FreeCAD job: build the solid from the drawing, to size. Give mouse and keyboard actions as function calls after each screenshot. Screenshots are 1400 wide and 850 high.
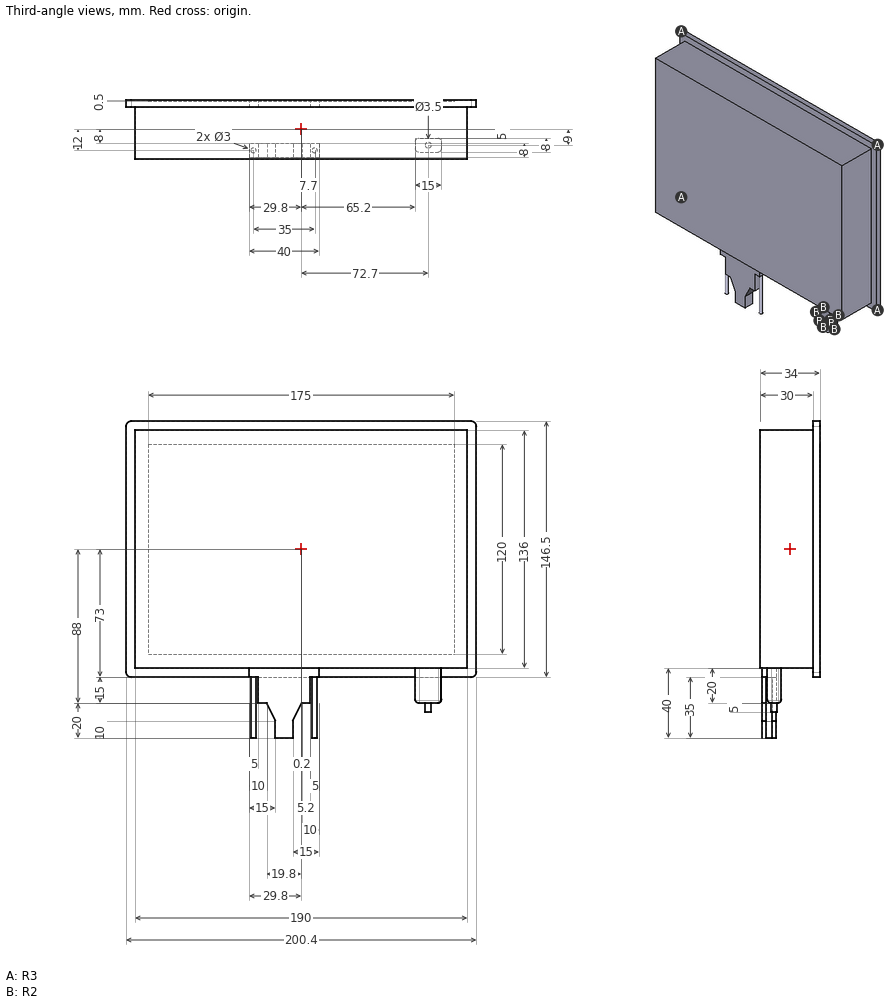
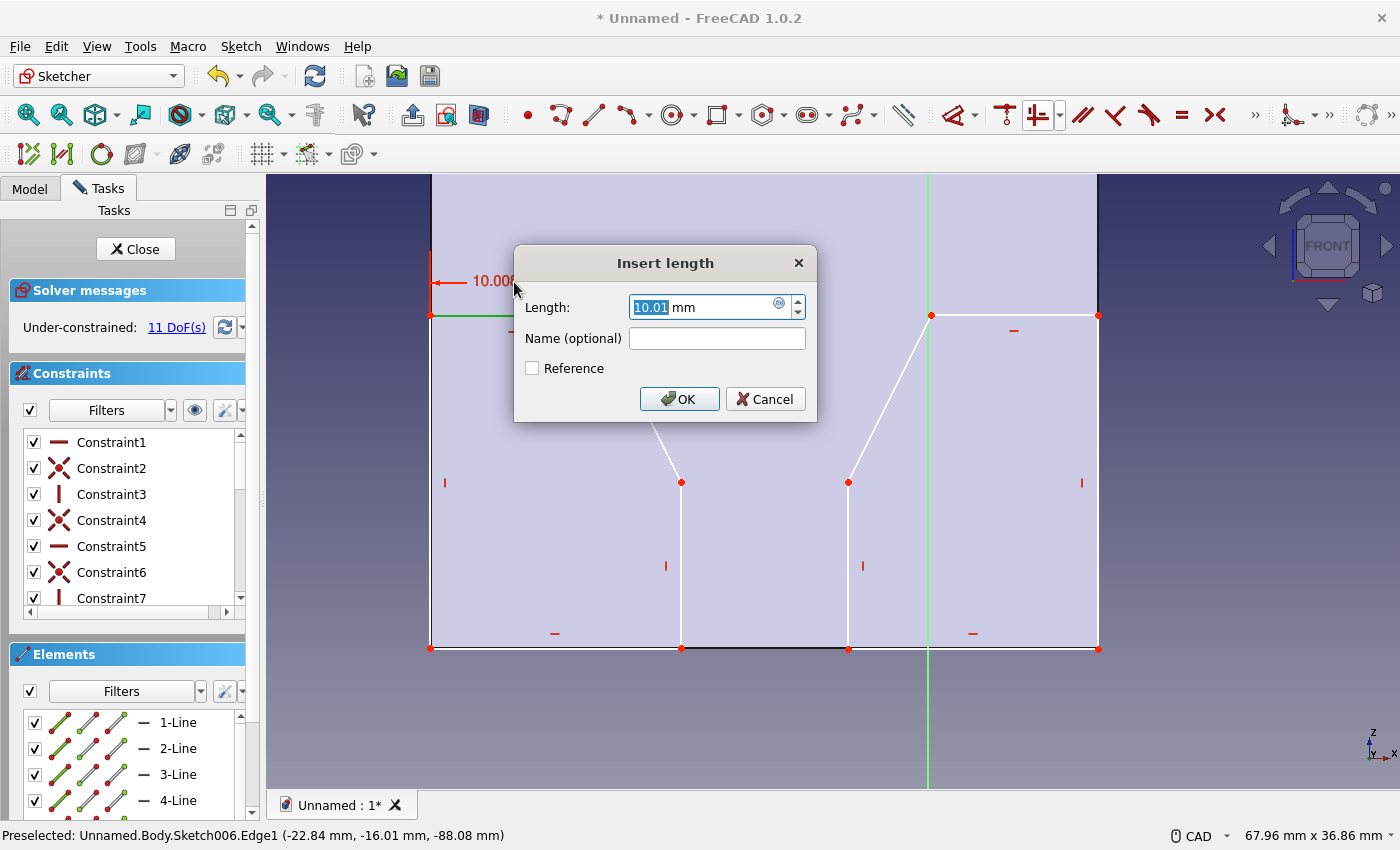
text(10)
key(Return)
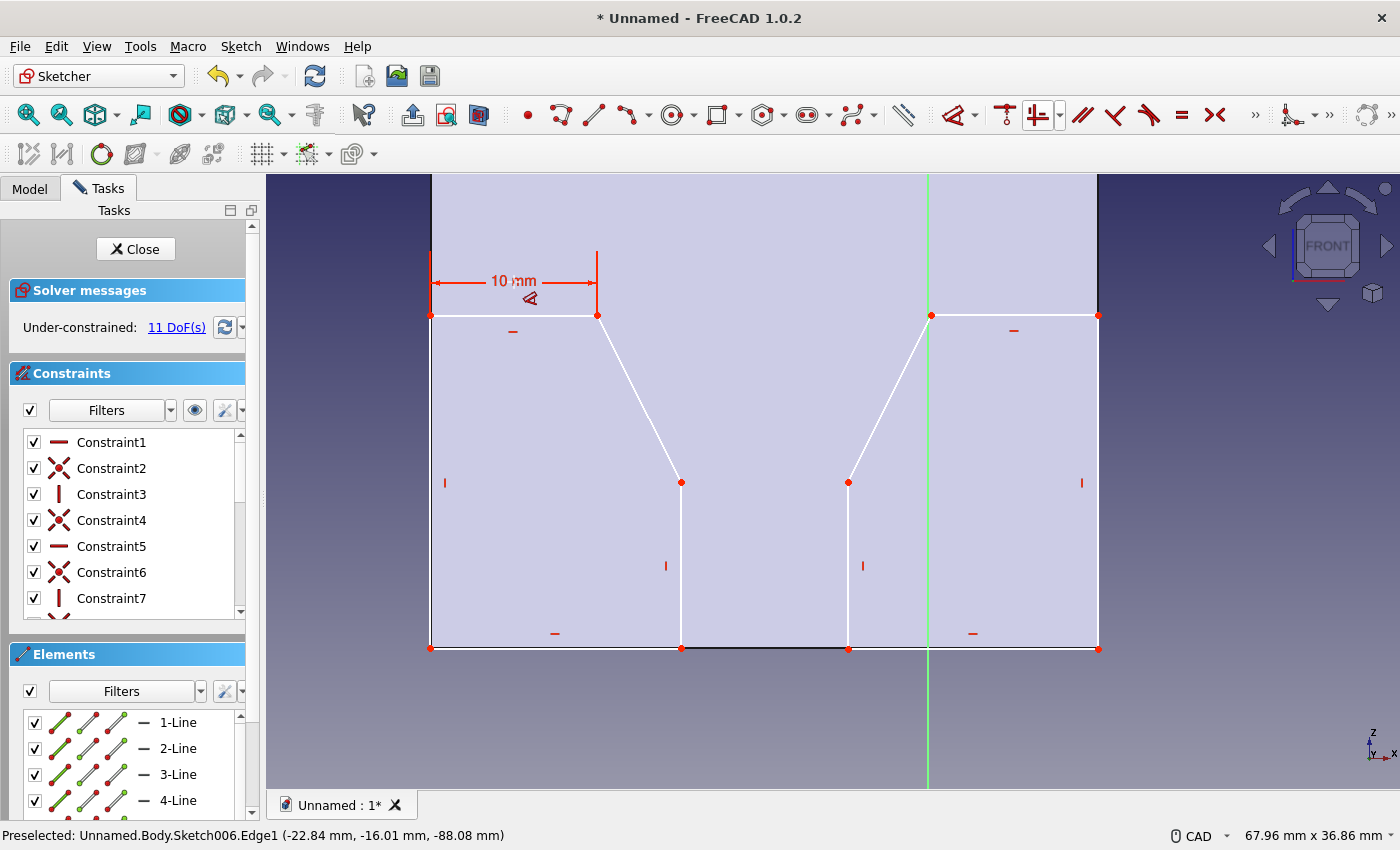
click(430, 416)
click(396, 482)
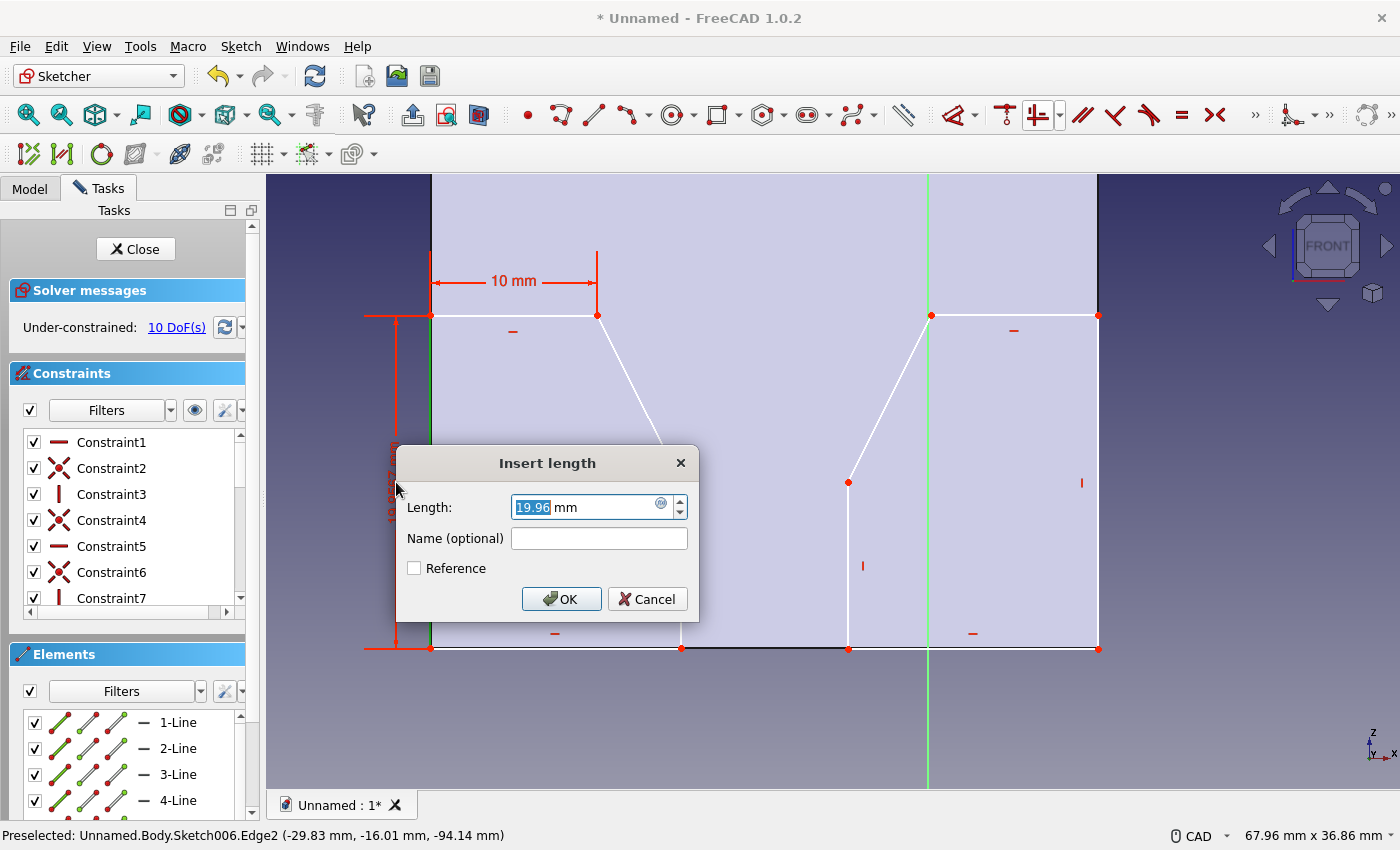
text(20)
key(Return)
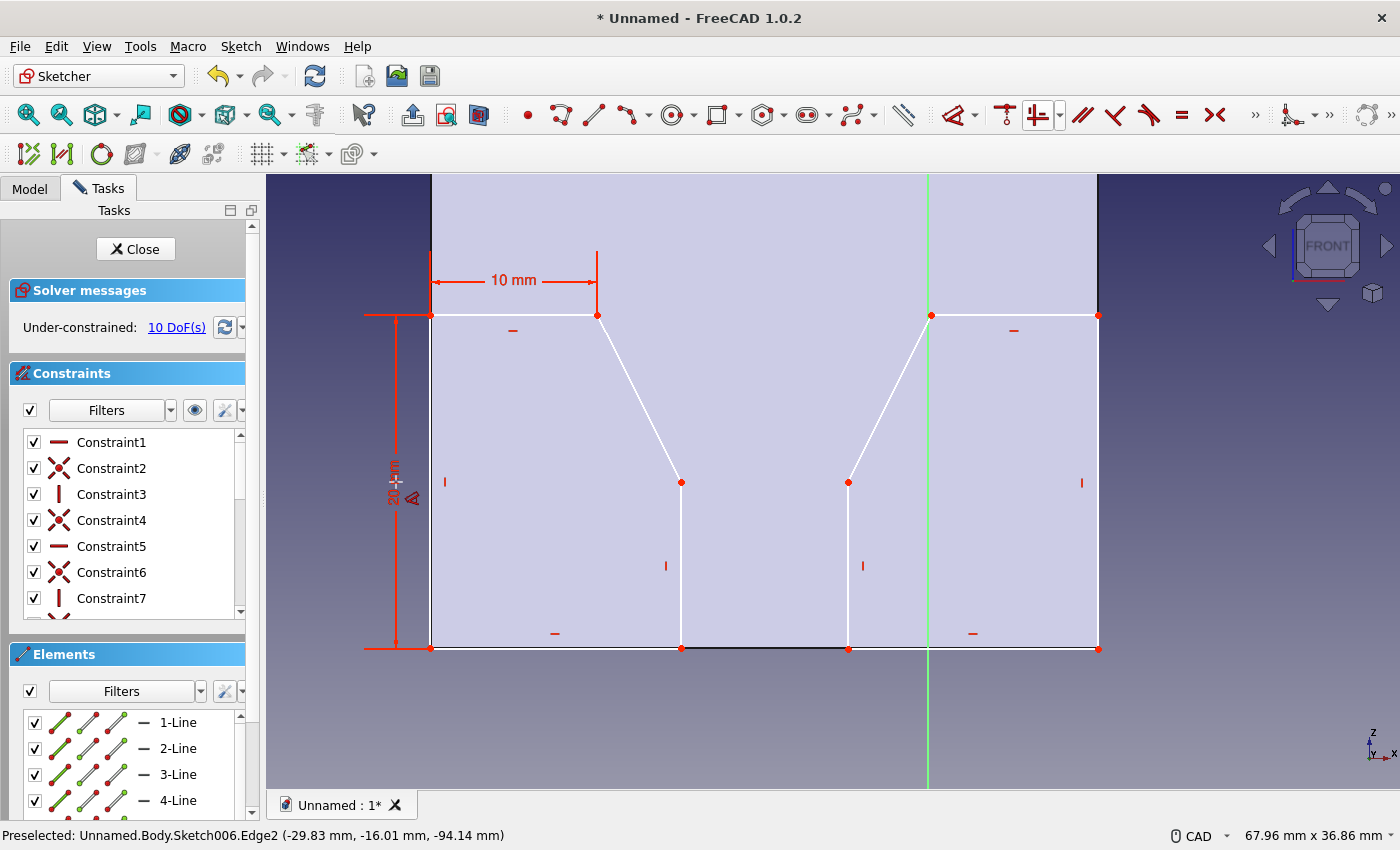
click(506, 649)
click(556, 683)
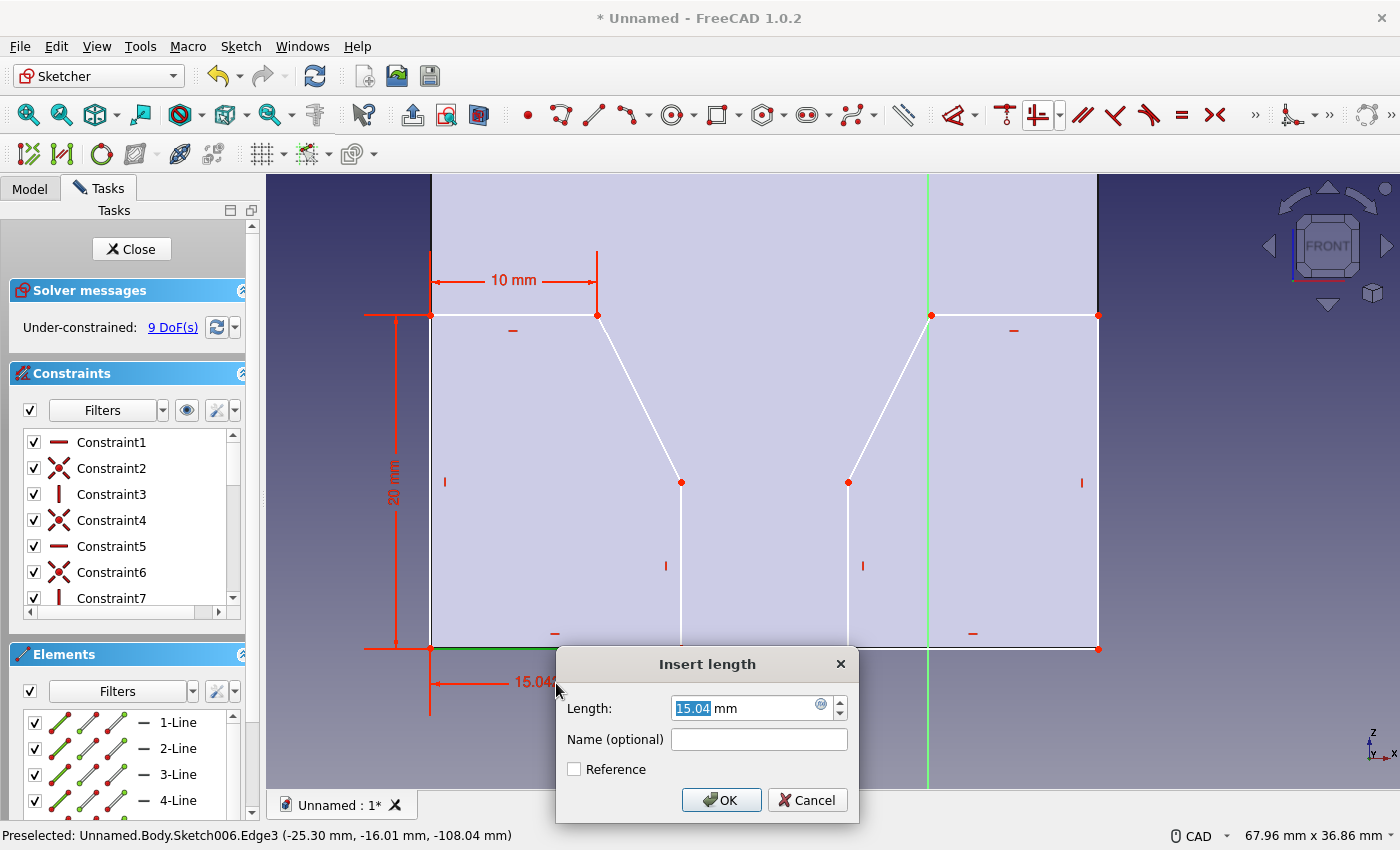
text(15)
key(Return)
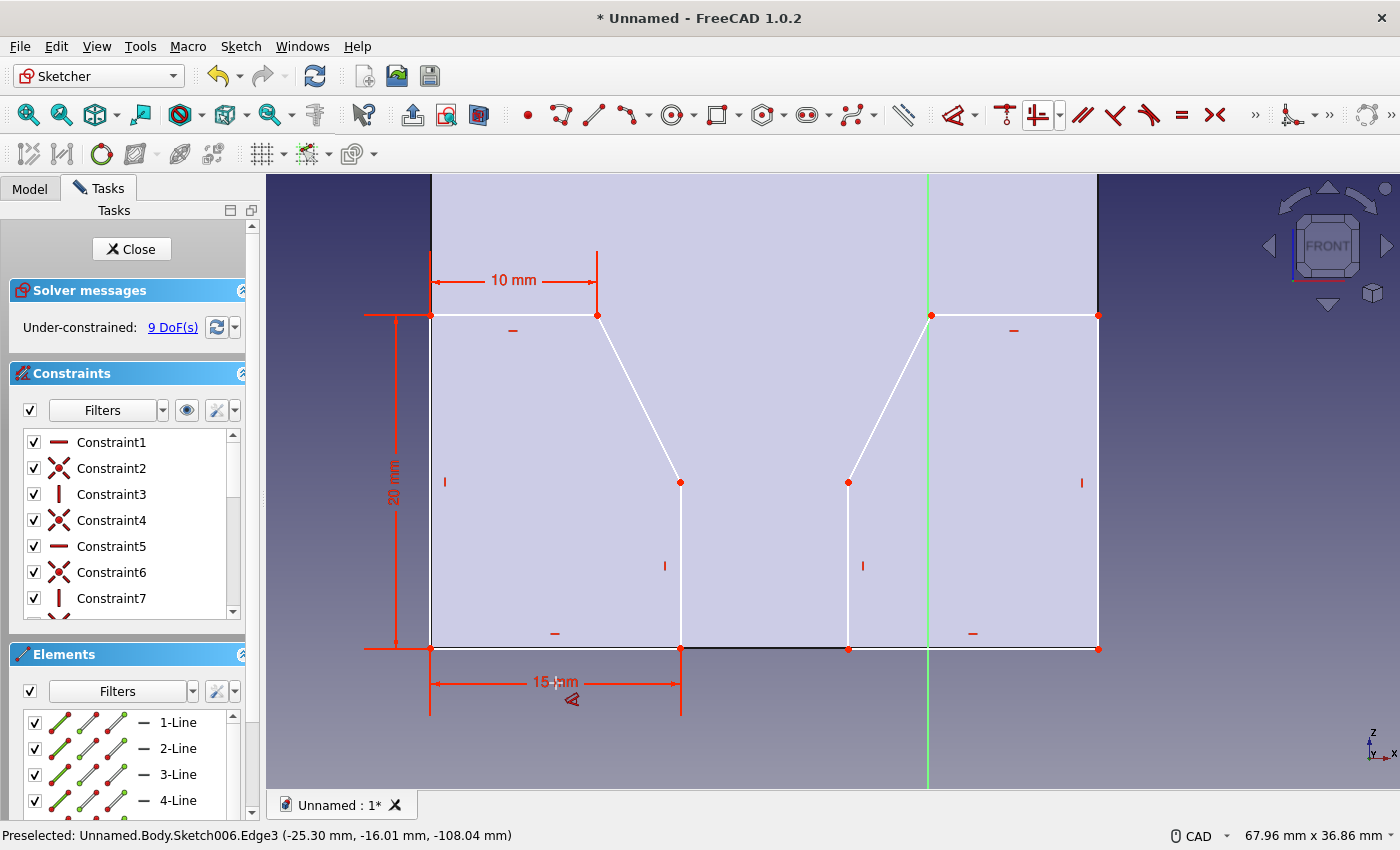
click(681, 599)
click(647, 566)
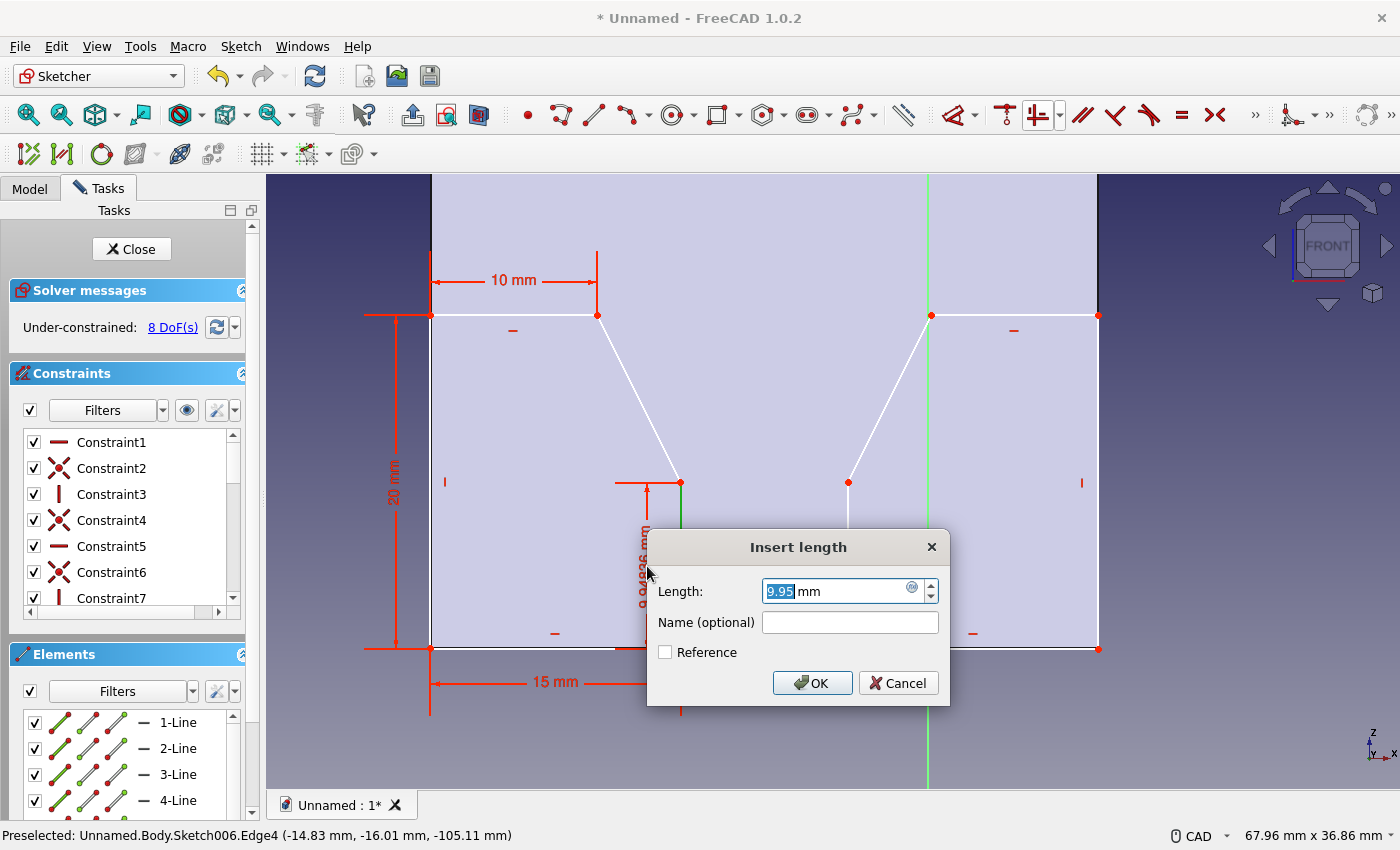
text(10)
key(Return)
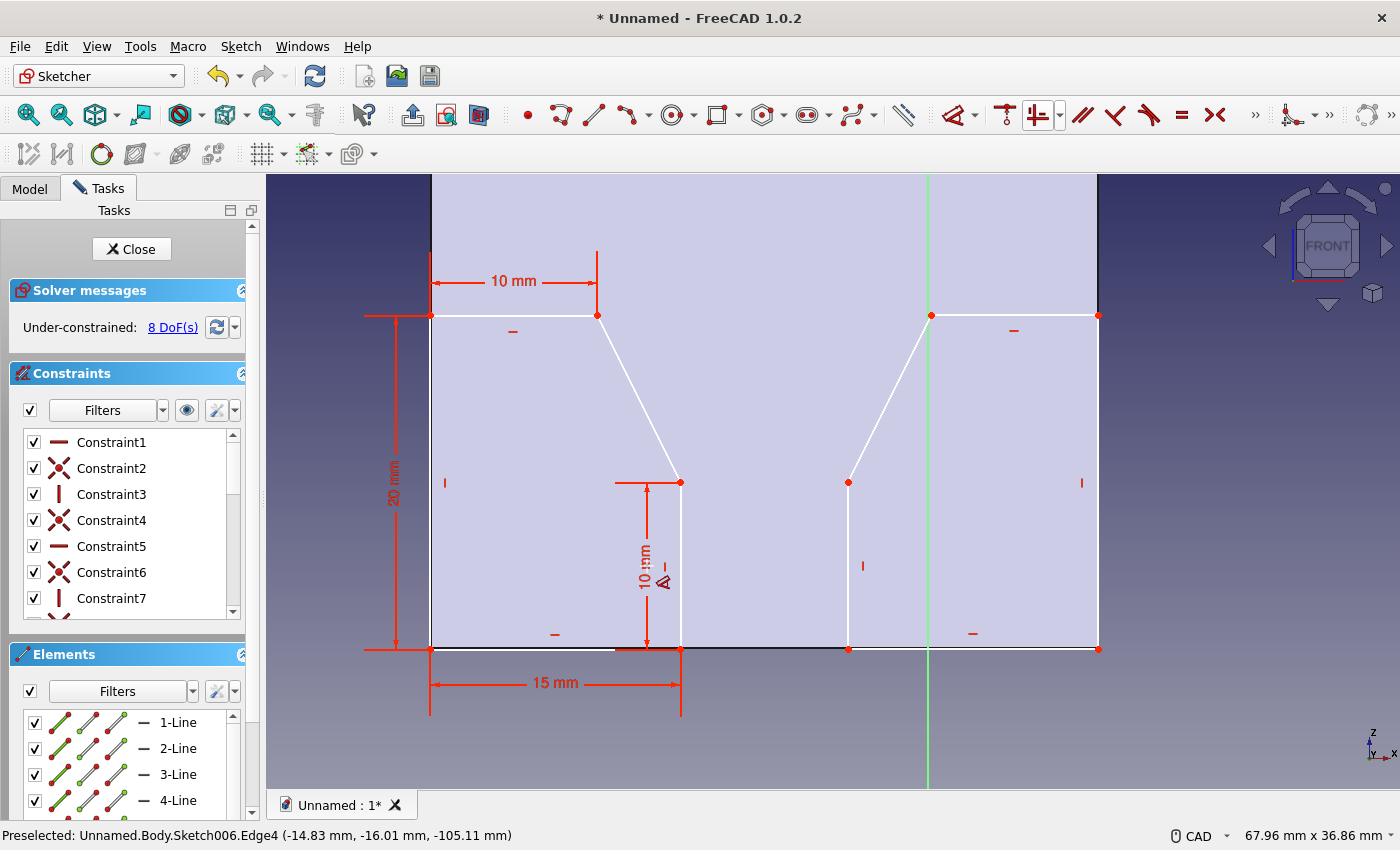
click(848, 532)
click(882, 566)